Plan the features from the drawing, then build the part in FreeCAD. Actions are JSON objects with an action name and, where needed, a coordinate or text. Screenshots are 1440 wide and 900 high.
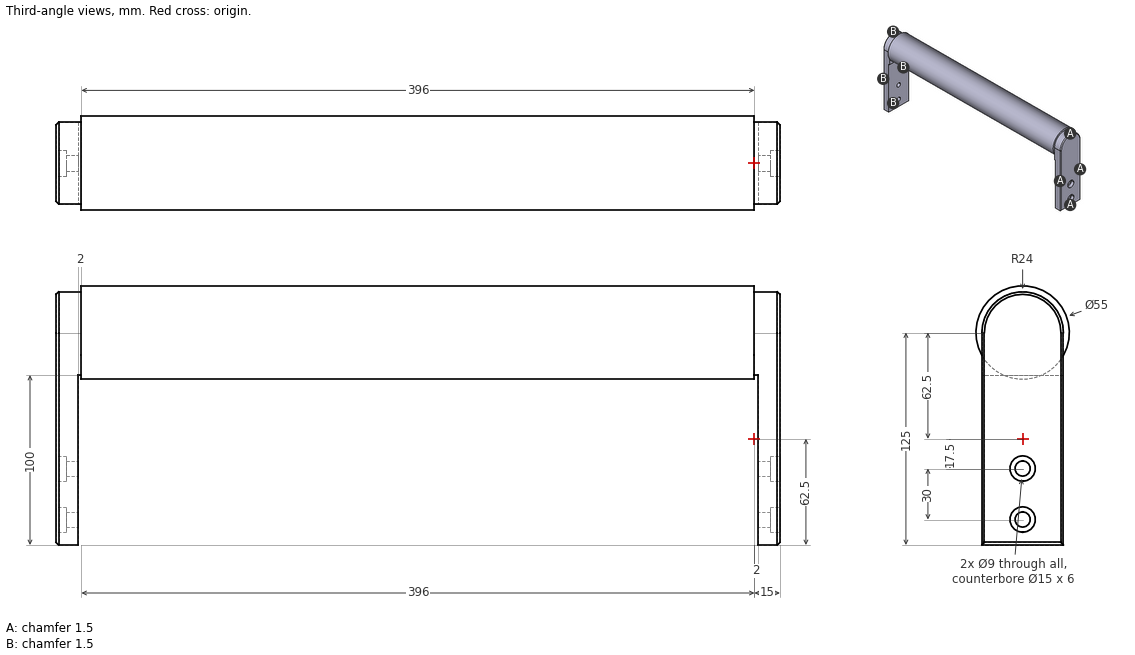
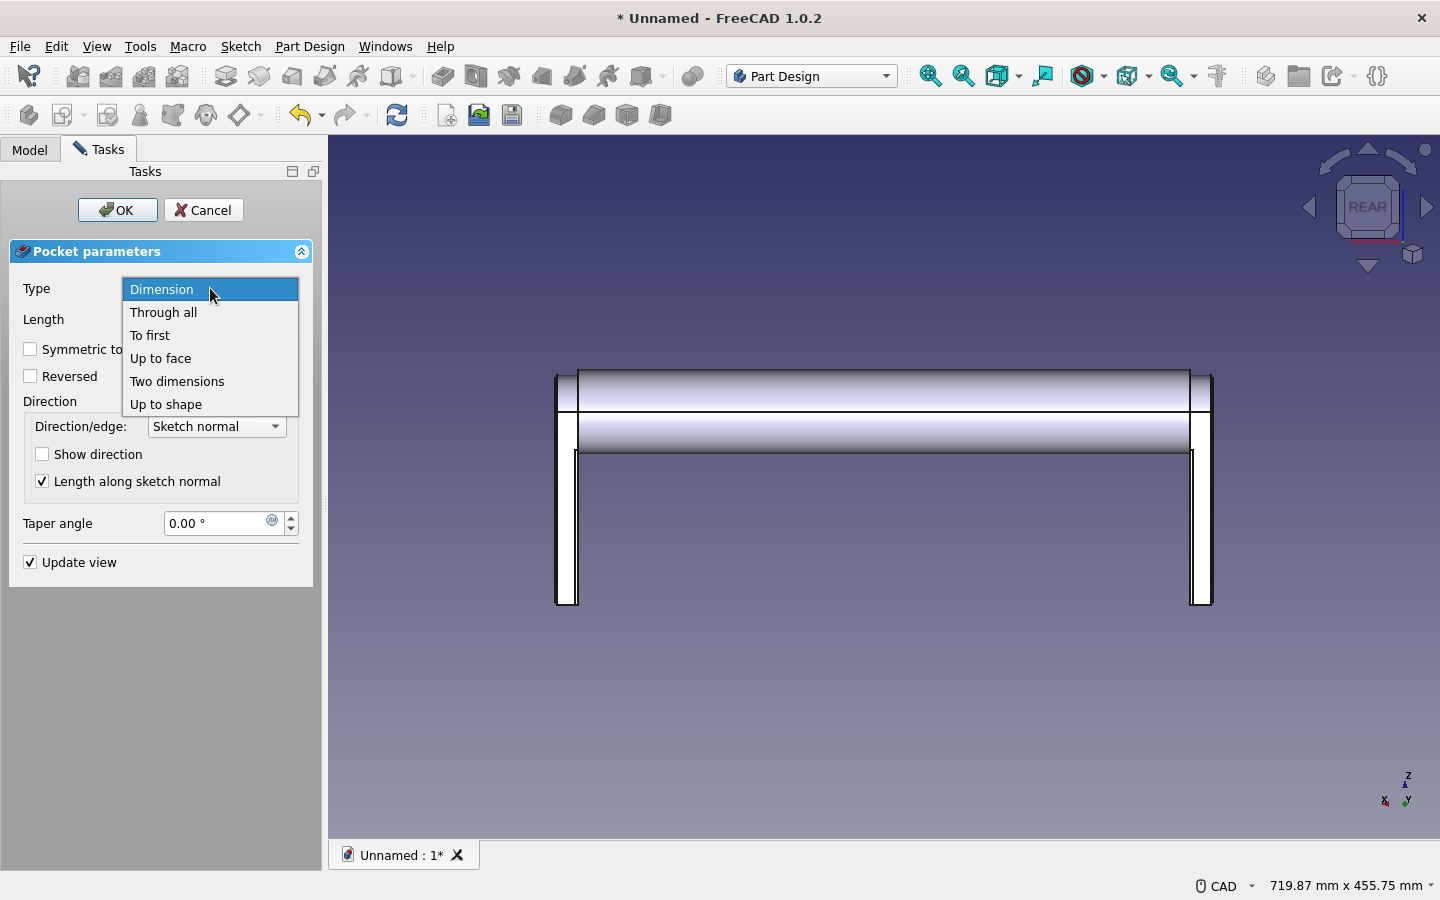
{"action": "left_click", "coordinate": [208, 312]}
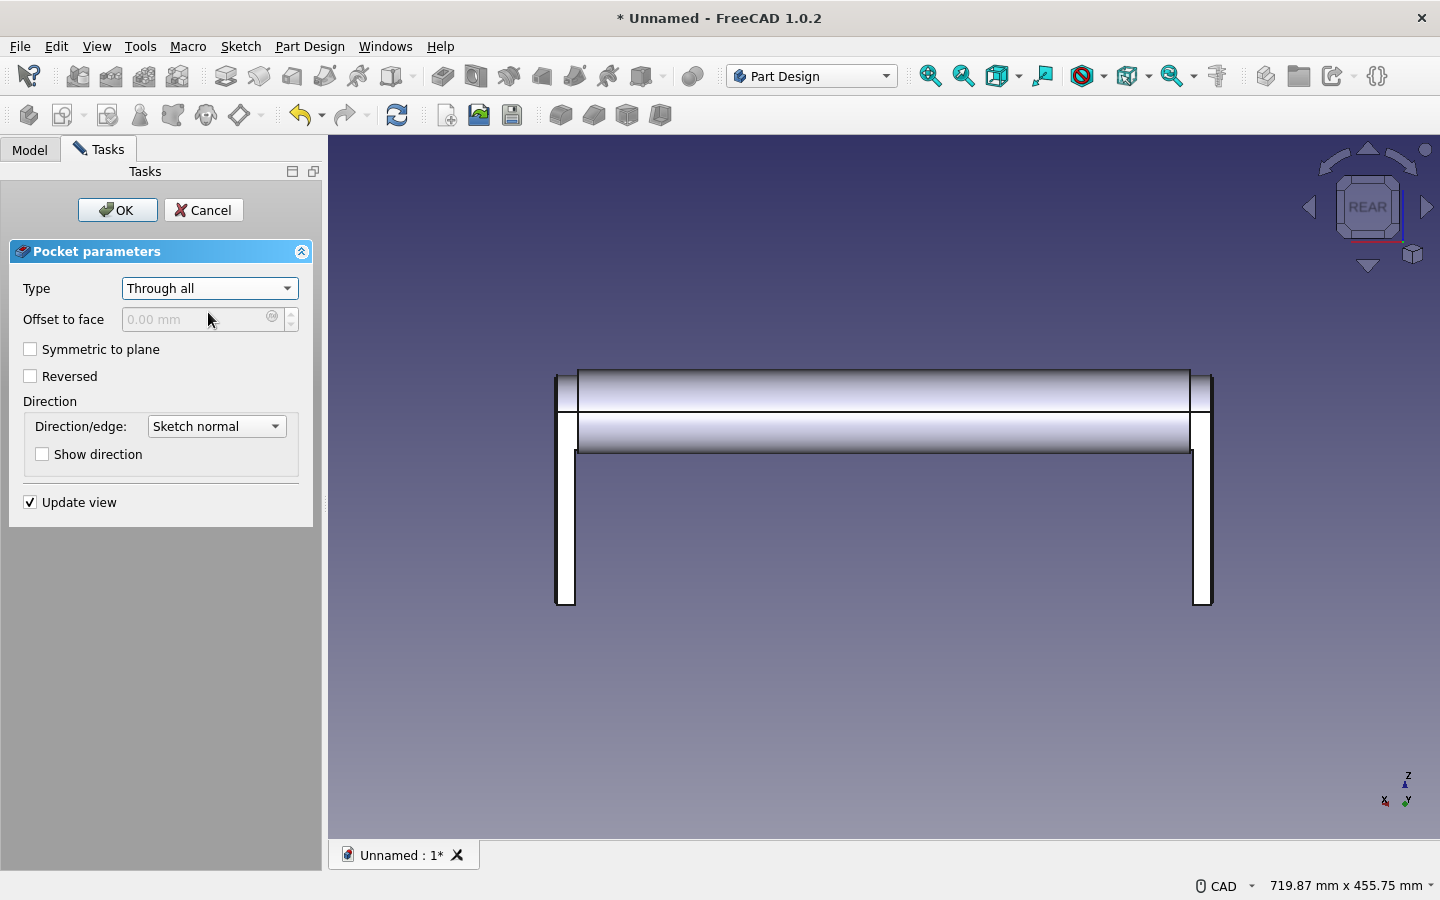
{"action": "left_click", "coordinate": [118, 210]}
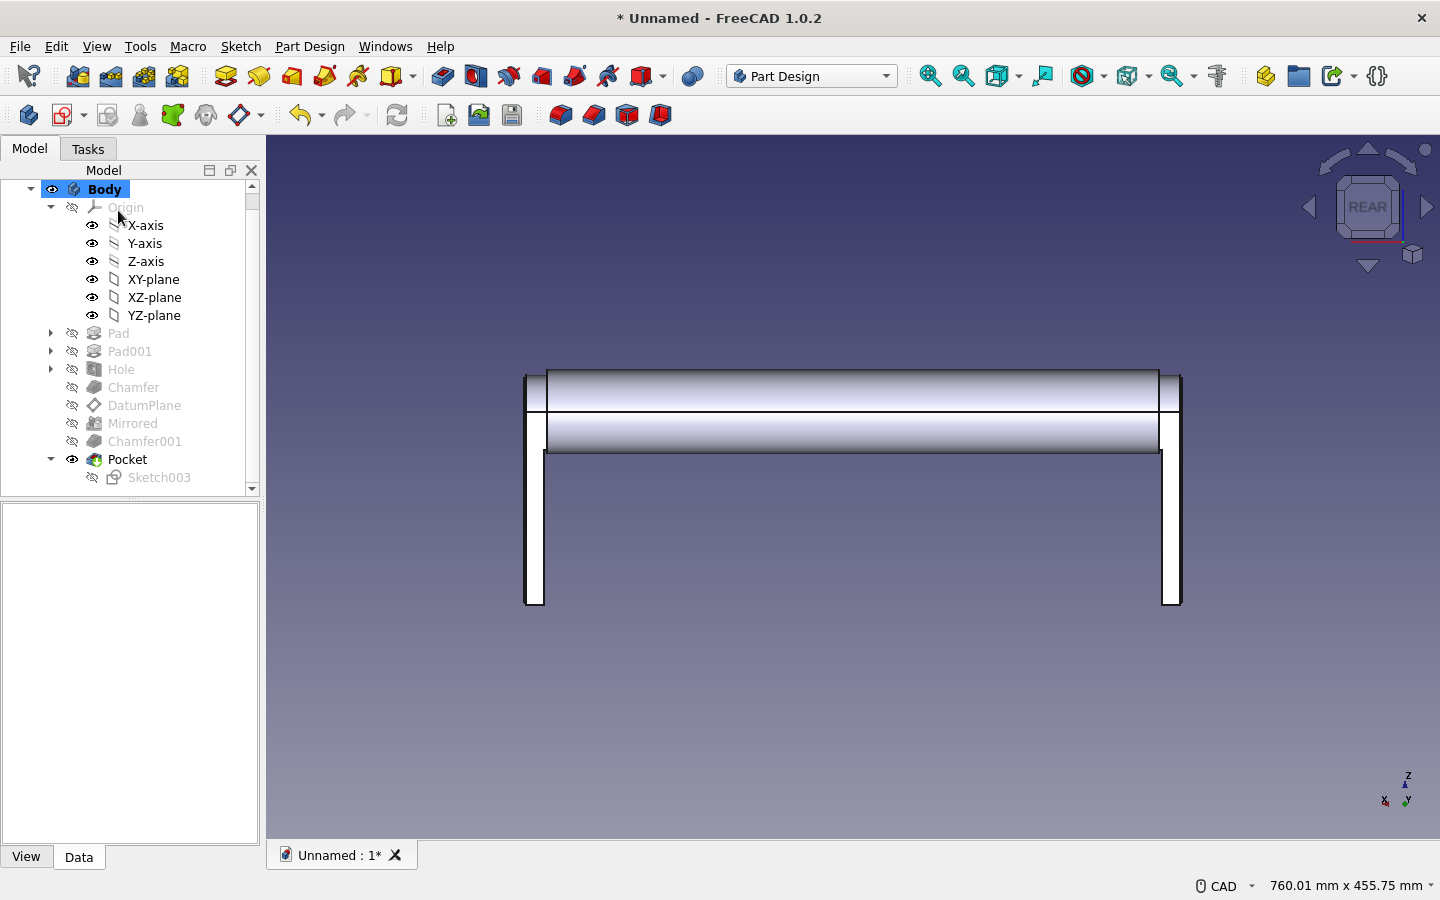
{"action": "key", "text": "0"}